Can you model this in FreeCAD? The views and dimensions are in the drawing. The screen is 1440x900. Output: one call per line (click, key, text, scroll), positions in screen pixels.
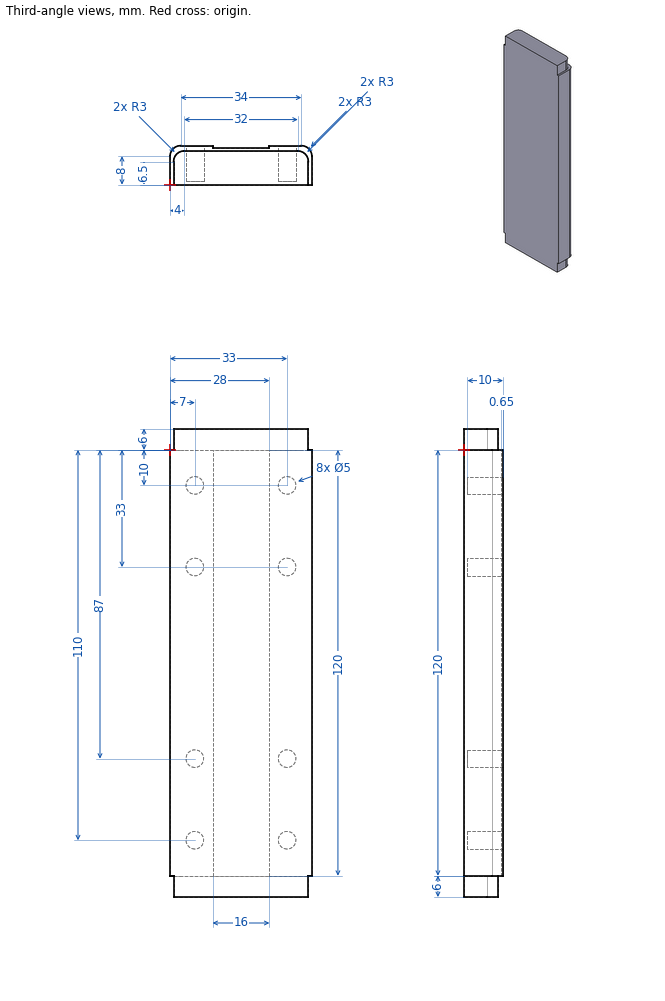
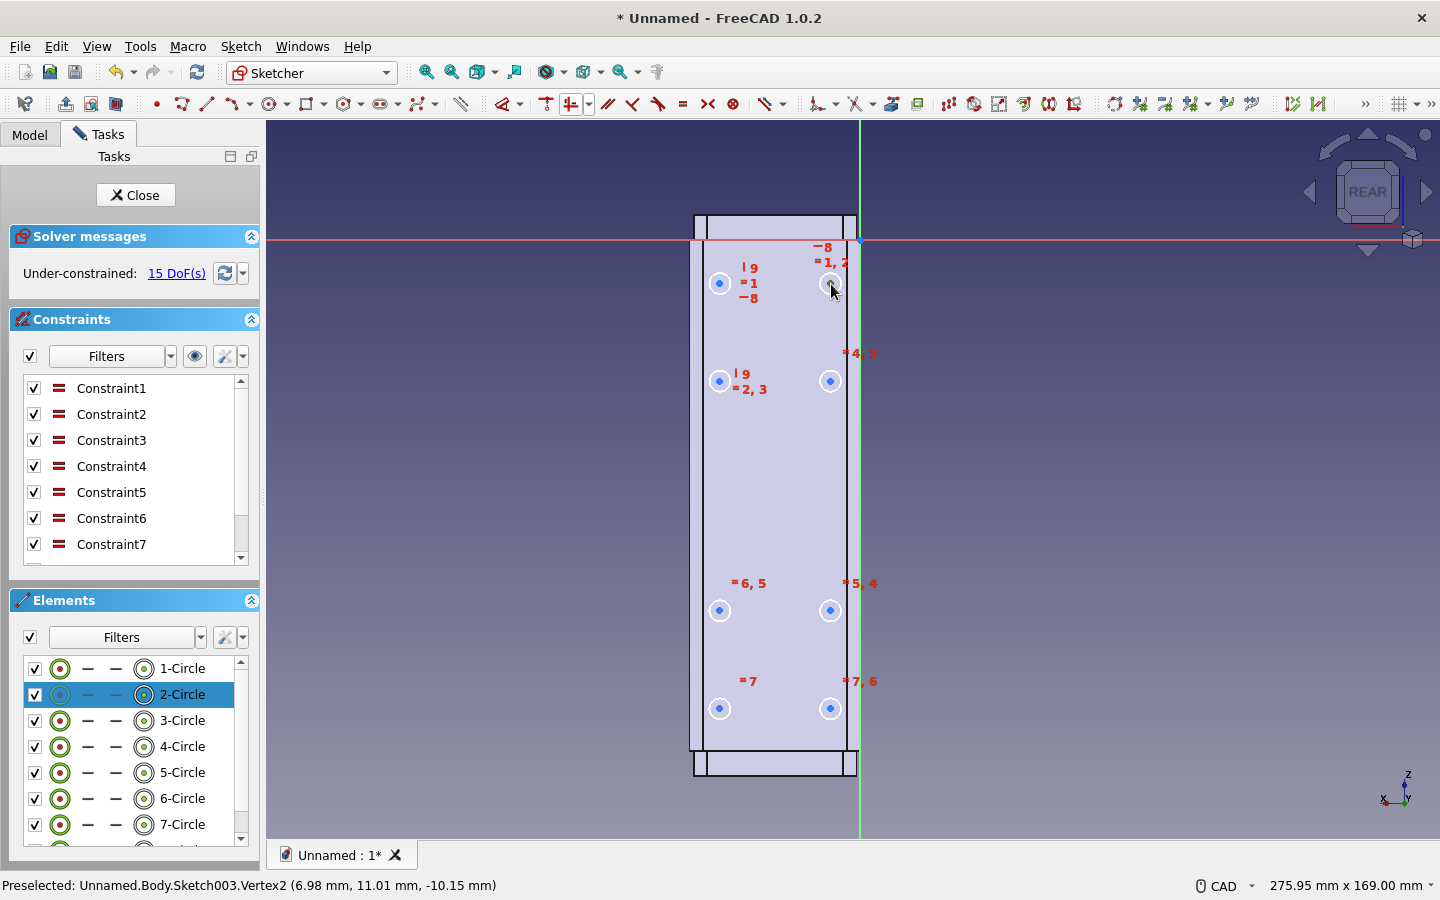
click(831, 381)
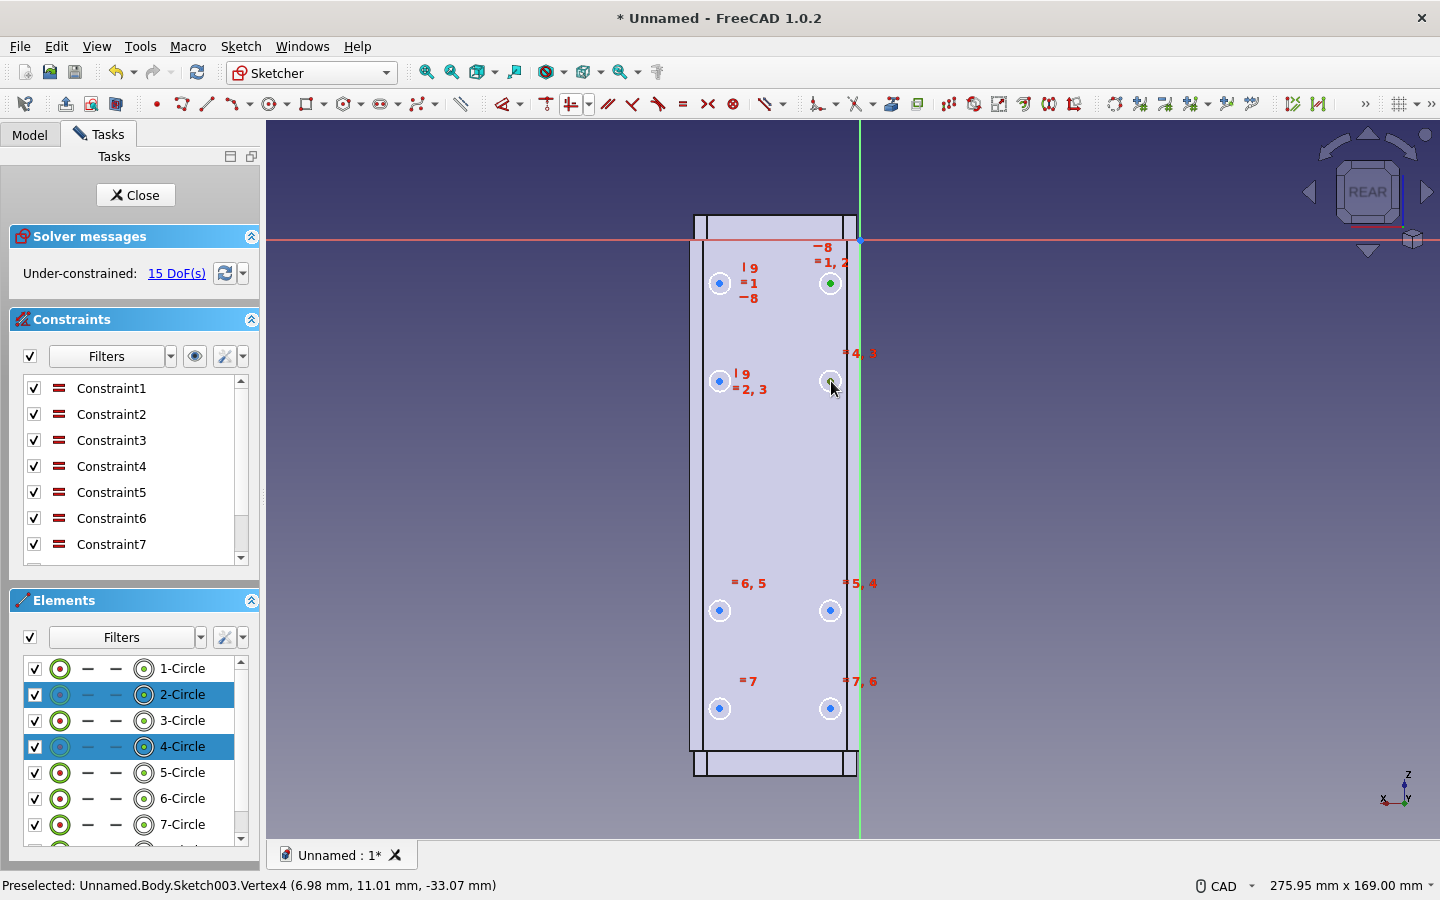
key(v)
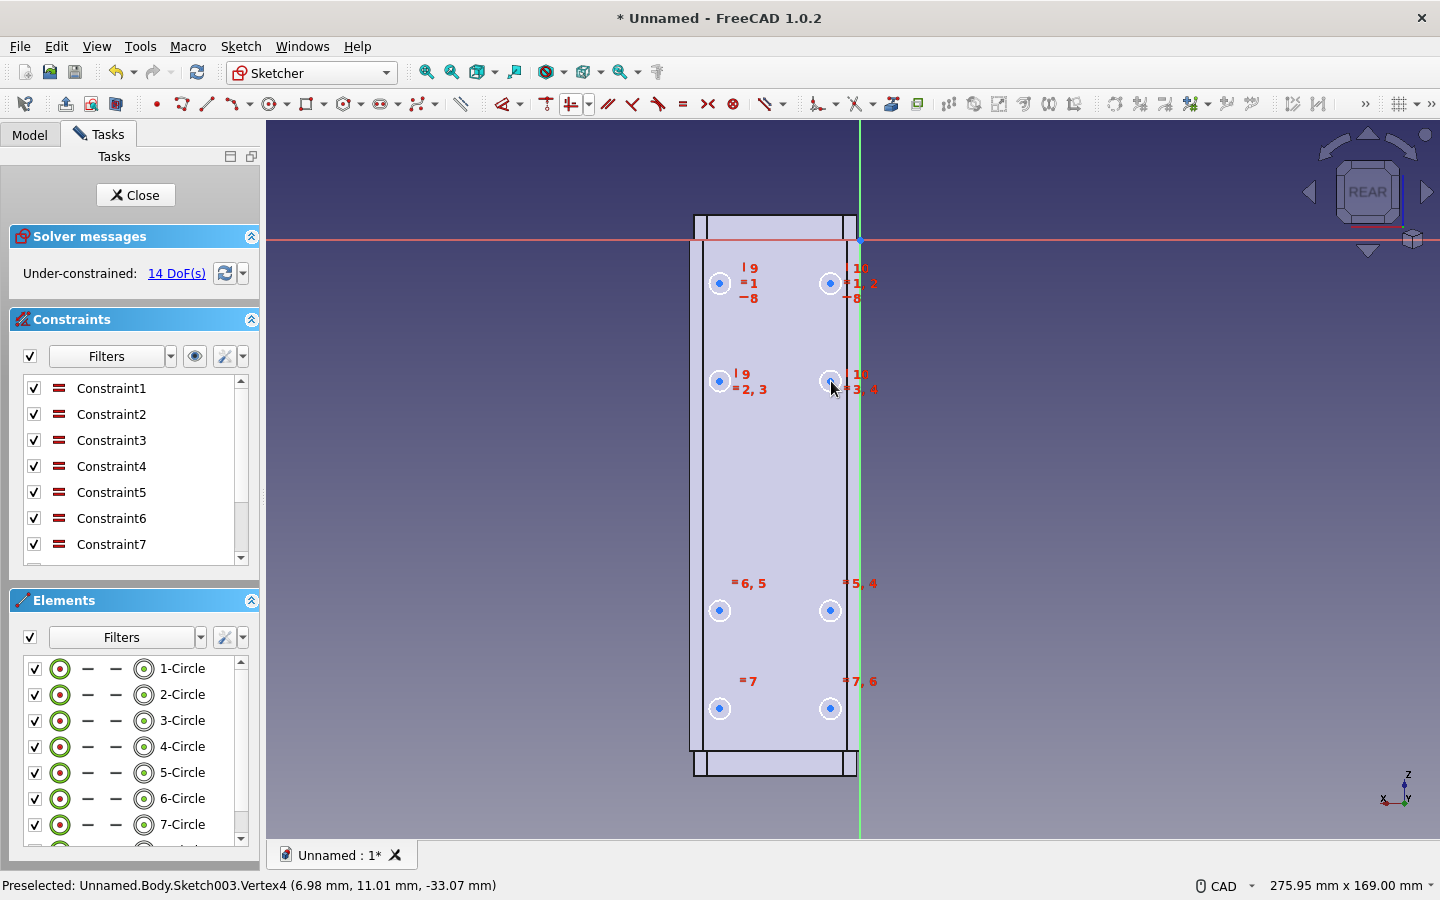
click(720, 381)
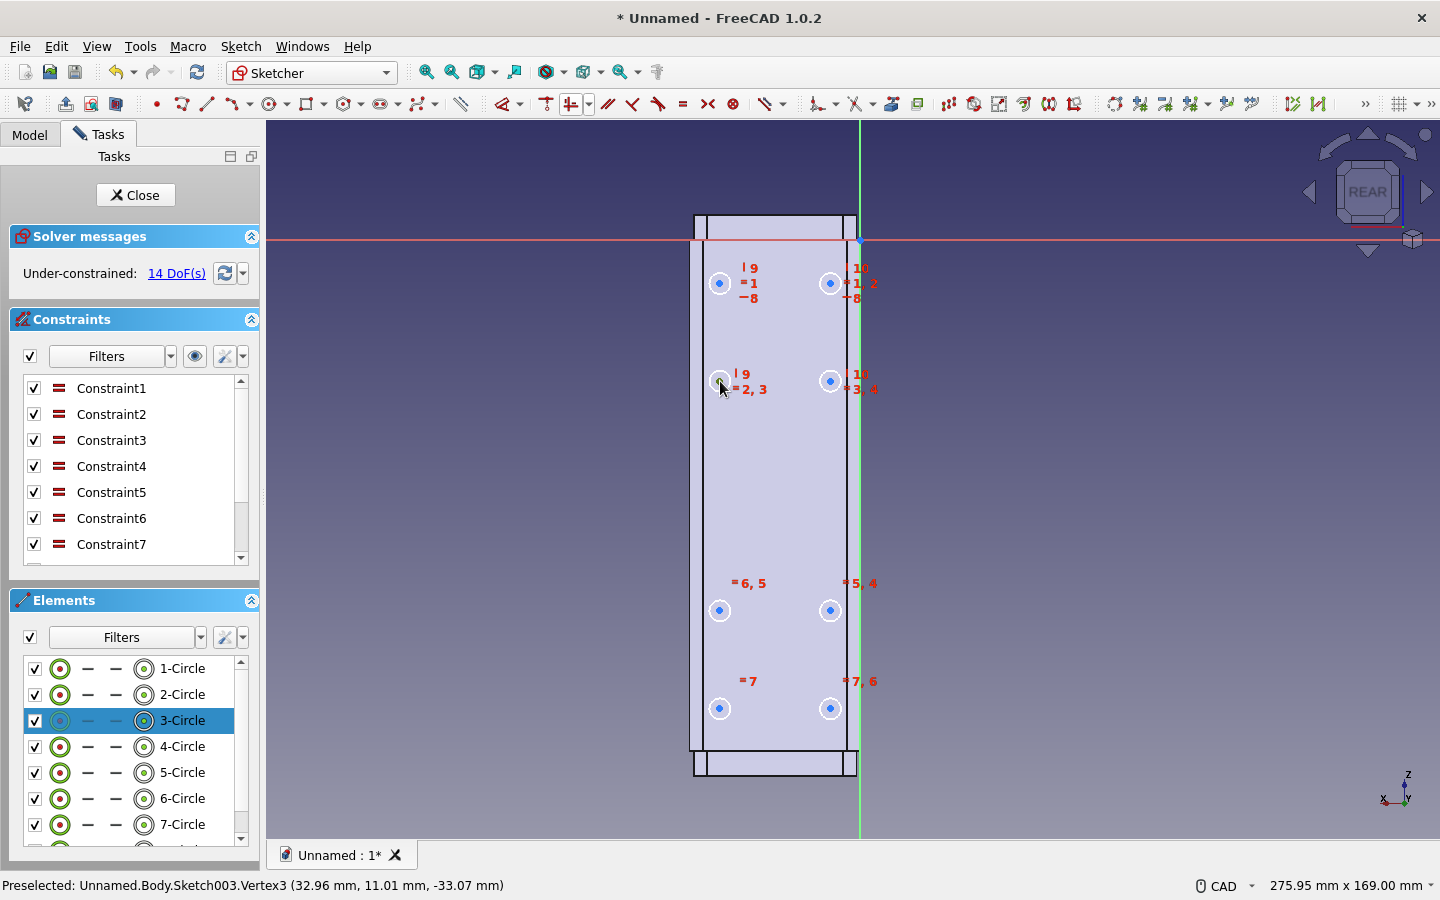
click(831, 381)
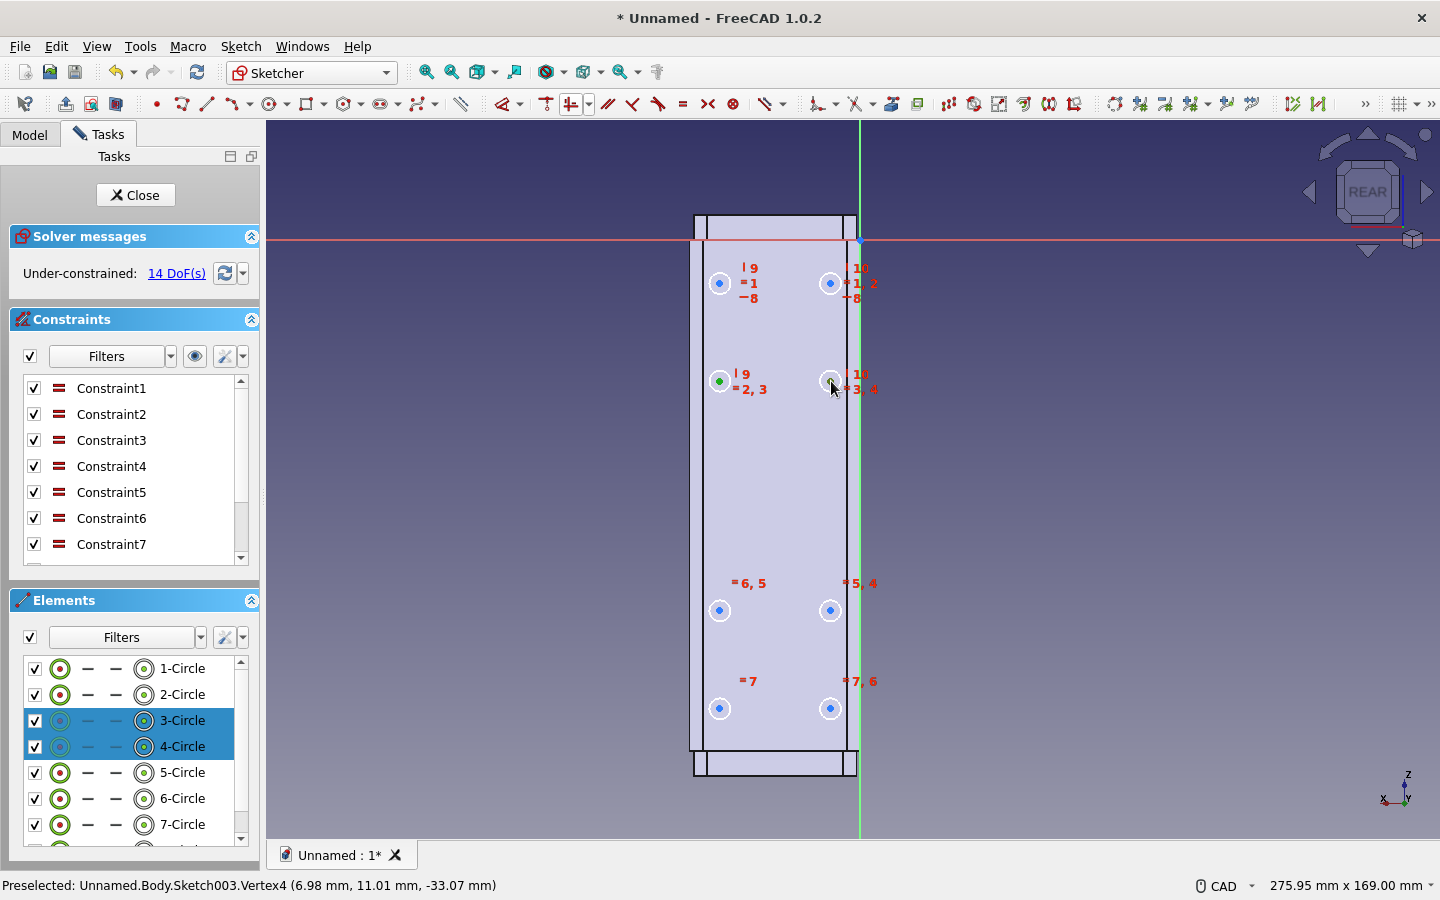
click(588, 104)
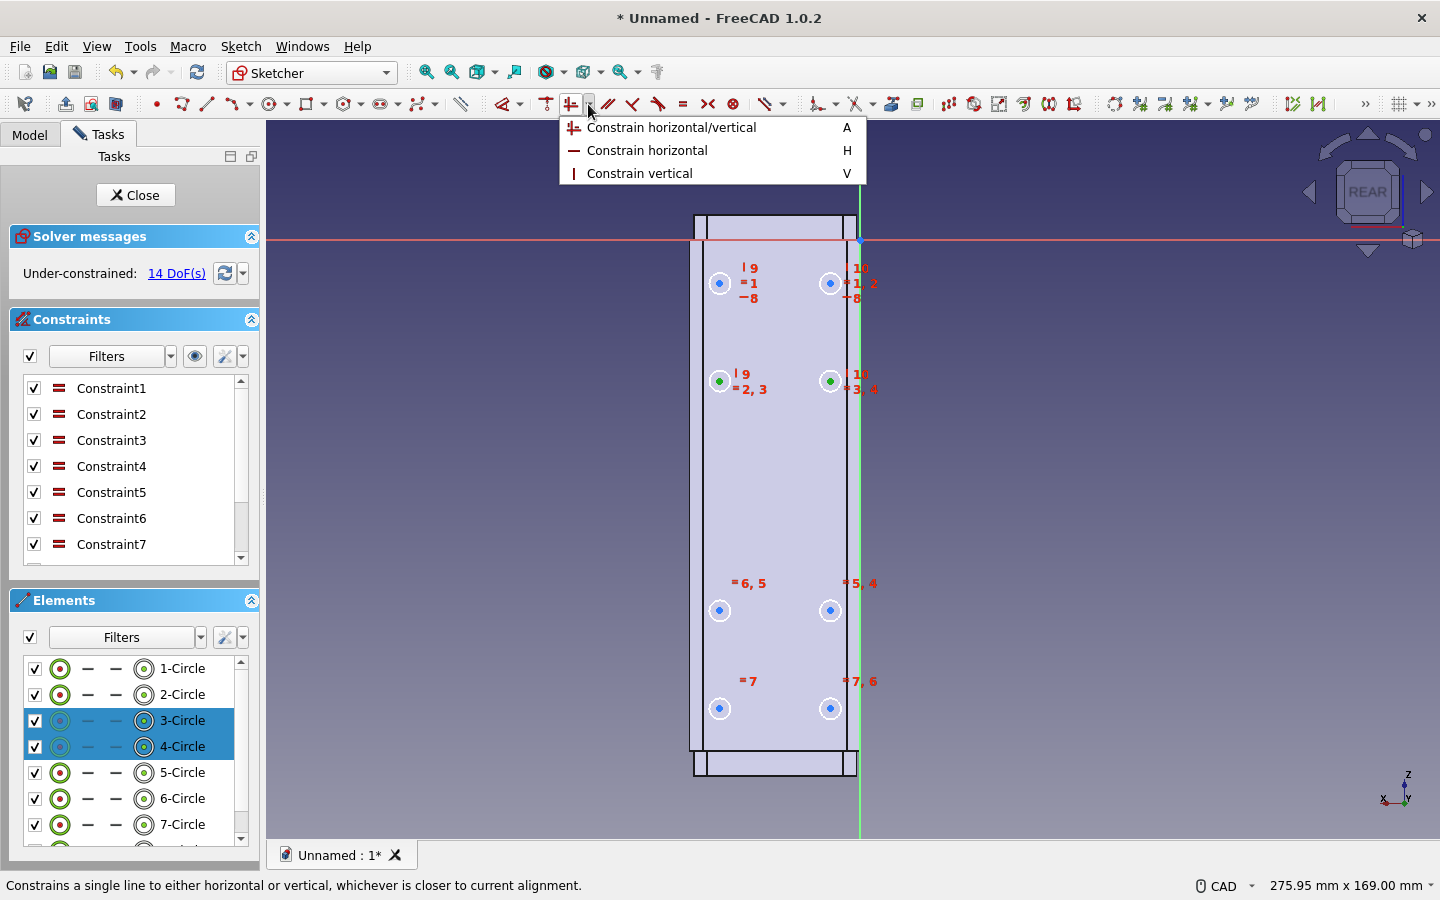
click(713, 150)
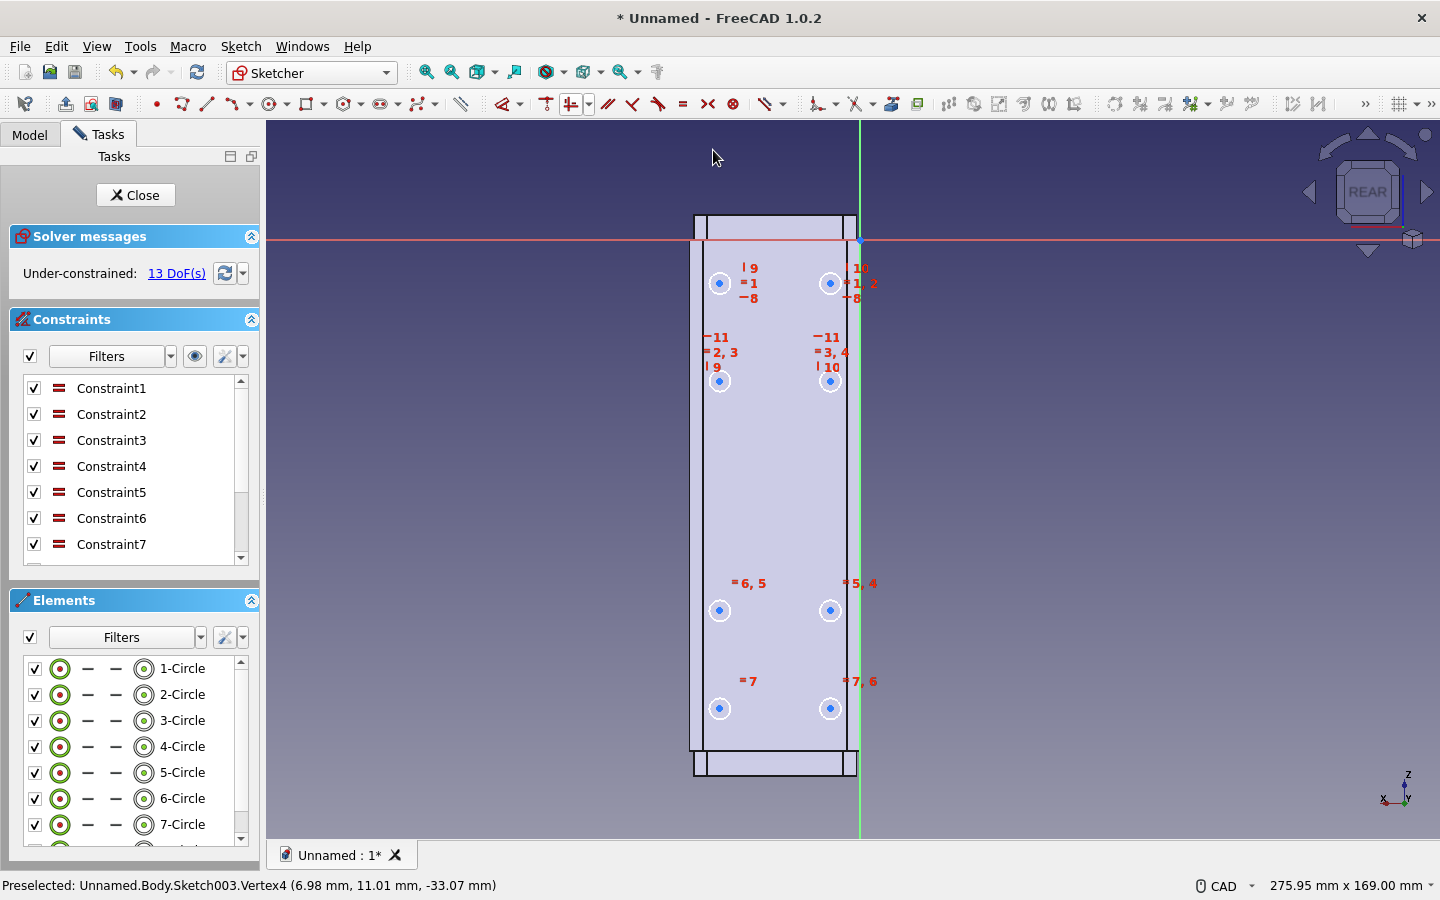
click(831, 381)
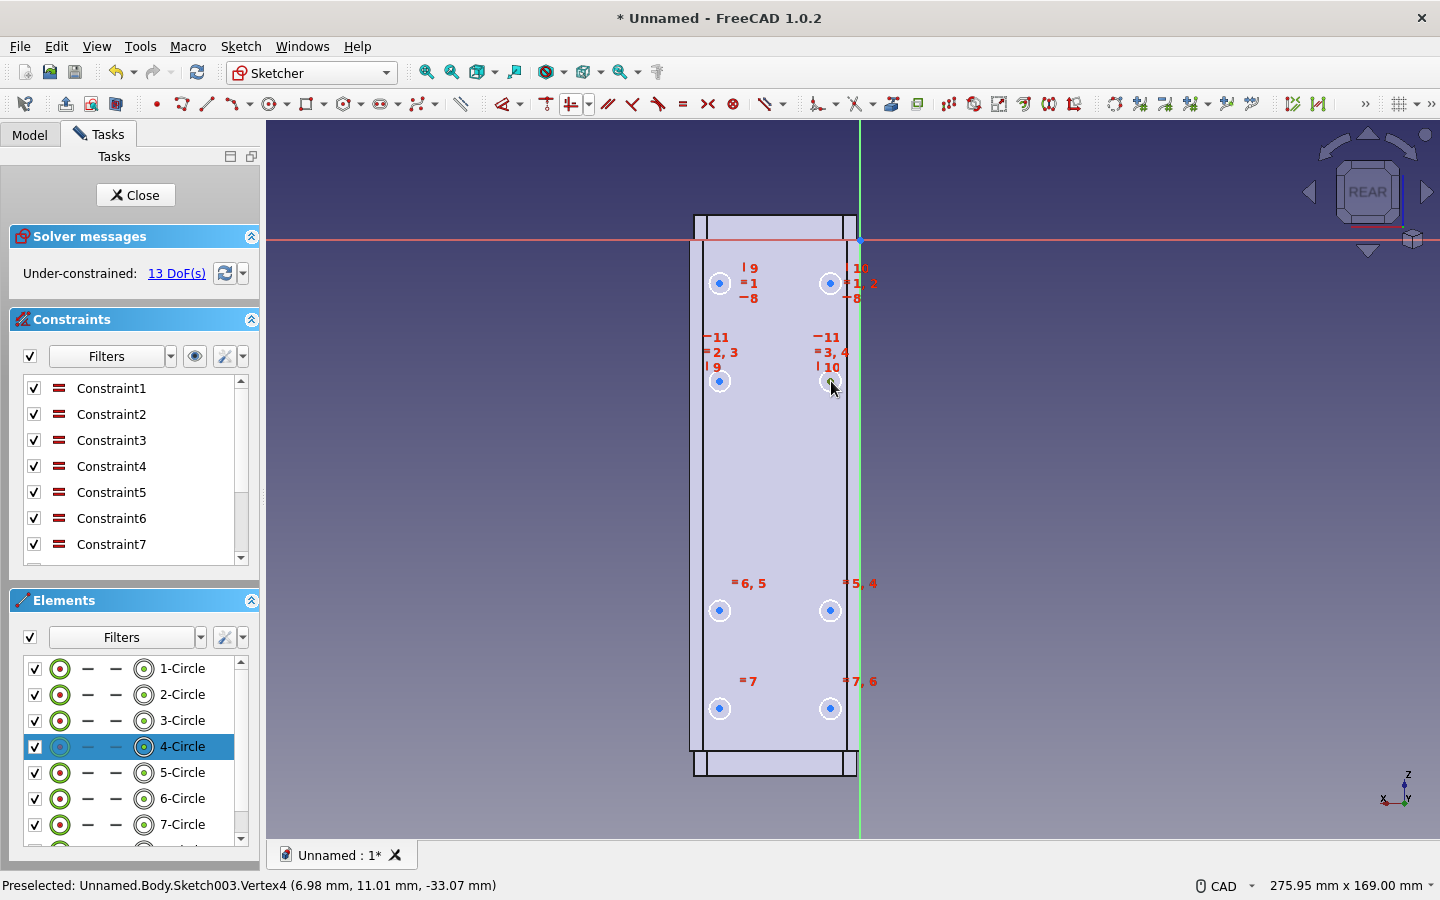
click(830, 611)